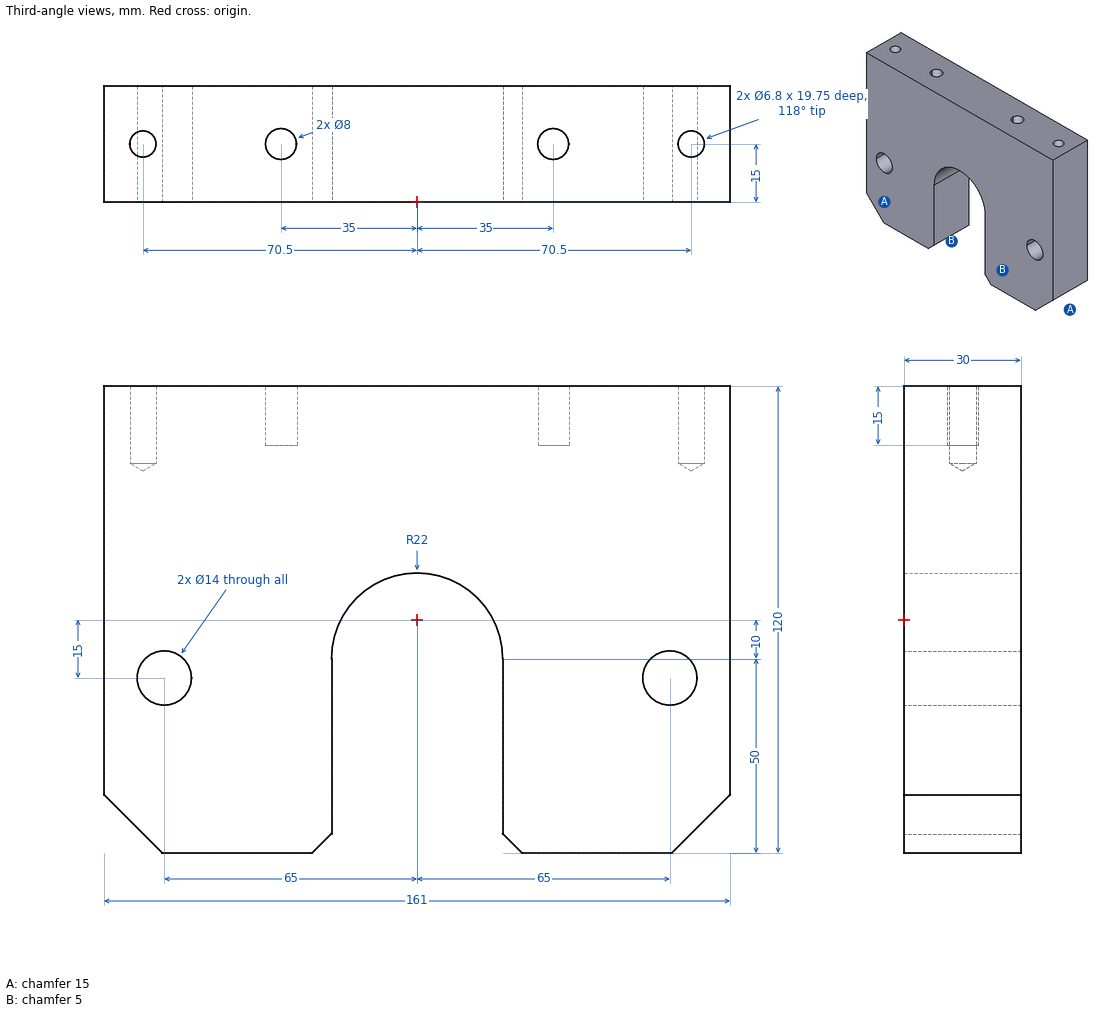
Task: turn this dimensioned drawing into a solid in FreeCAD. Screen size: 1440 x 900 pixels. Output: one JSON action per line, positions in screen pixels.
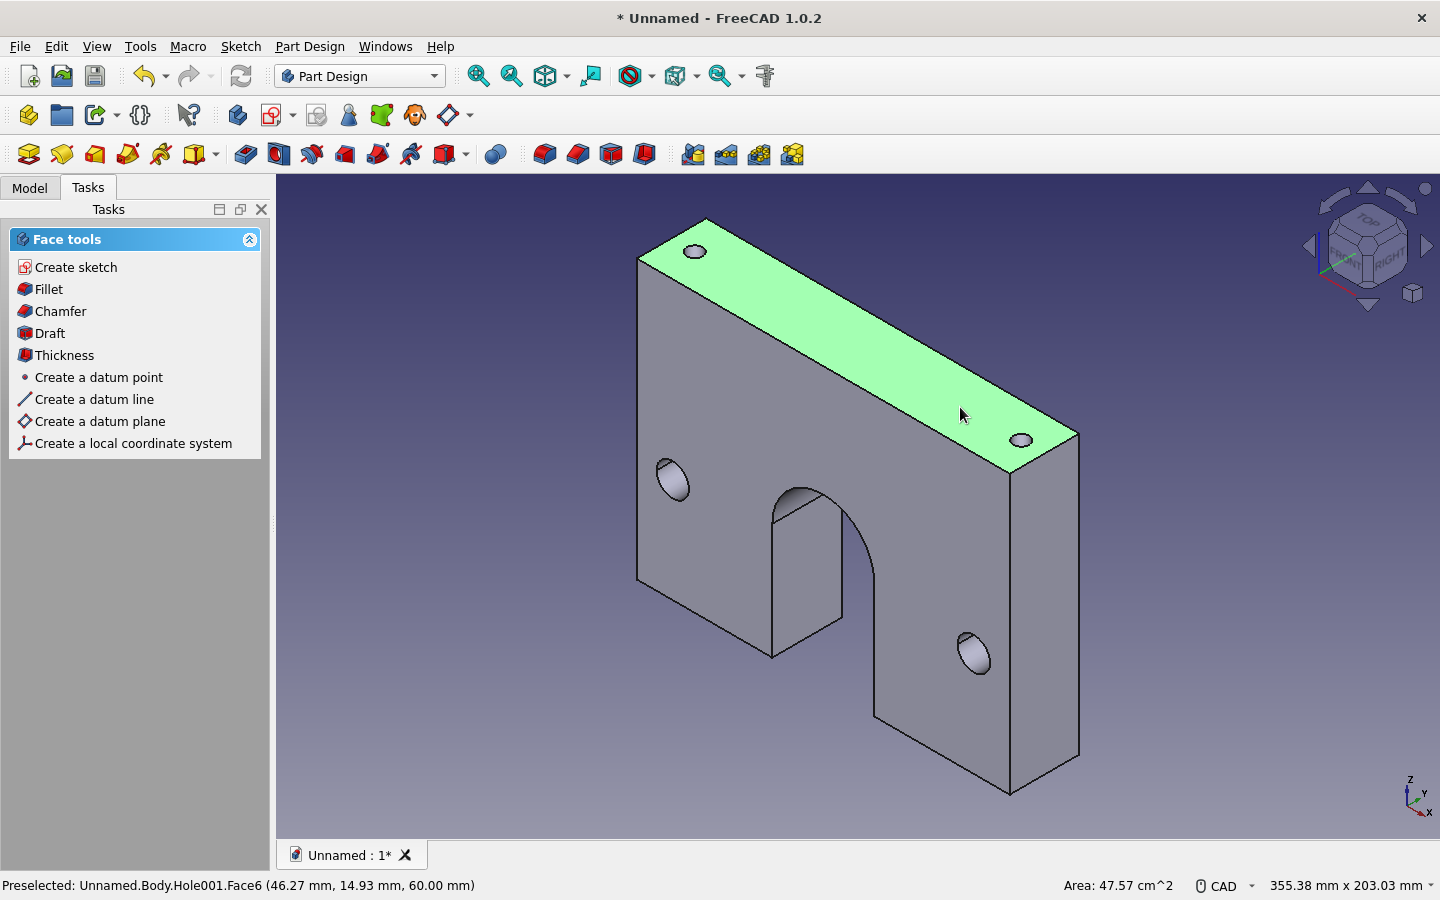
{"action": "left_click", "coordinate": [270, 116]}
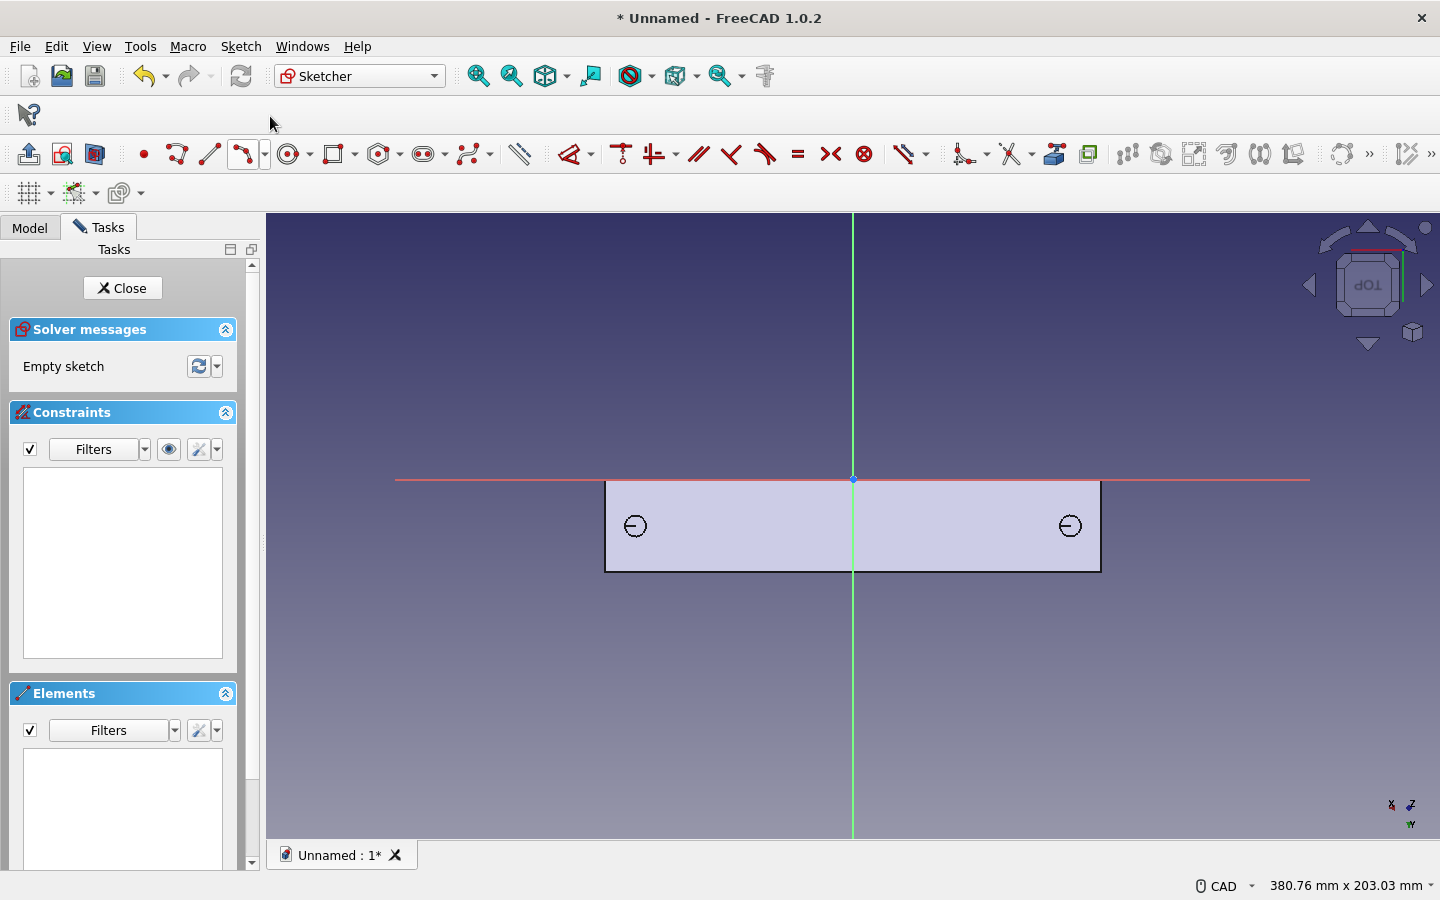
{"action": "scroll", "coordinate": [893, 499], "scroll_direction": "up", "scroll_amount": 5}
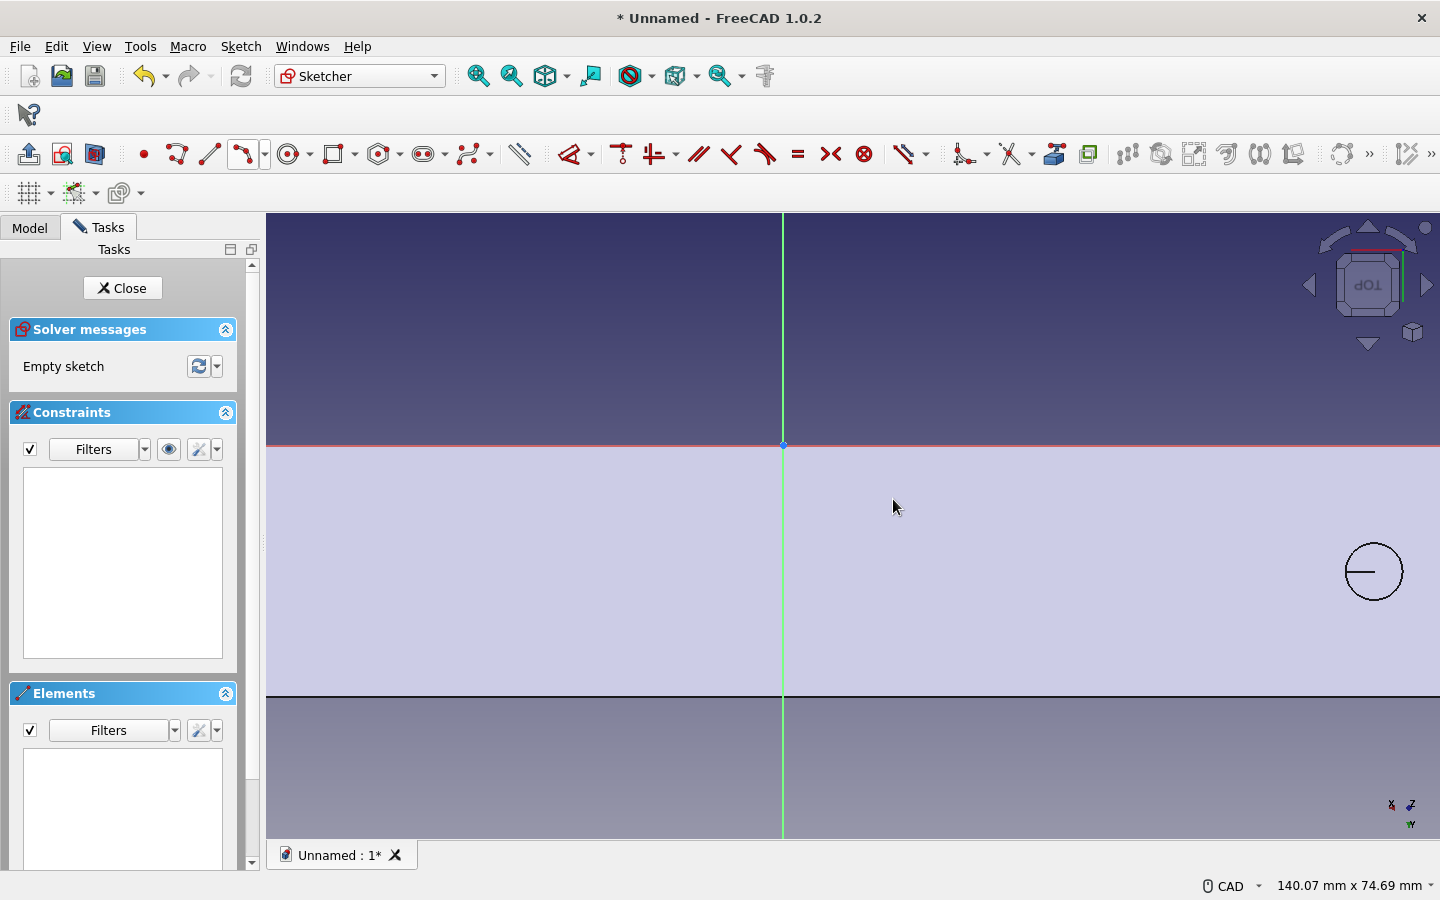
{"action": "key", "text": "g c"}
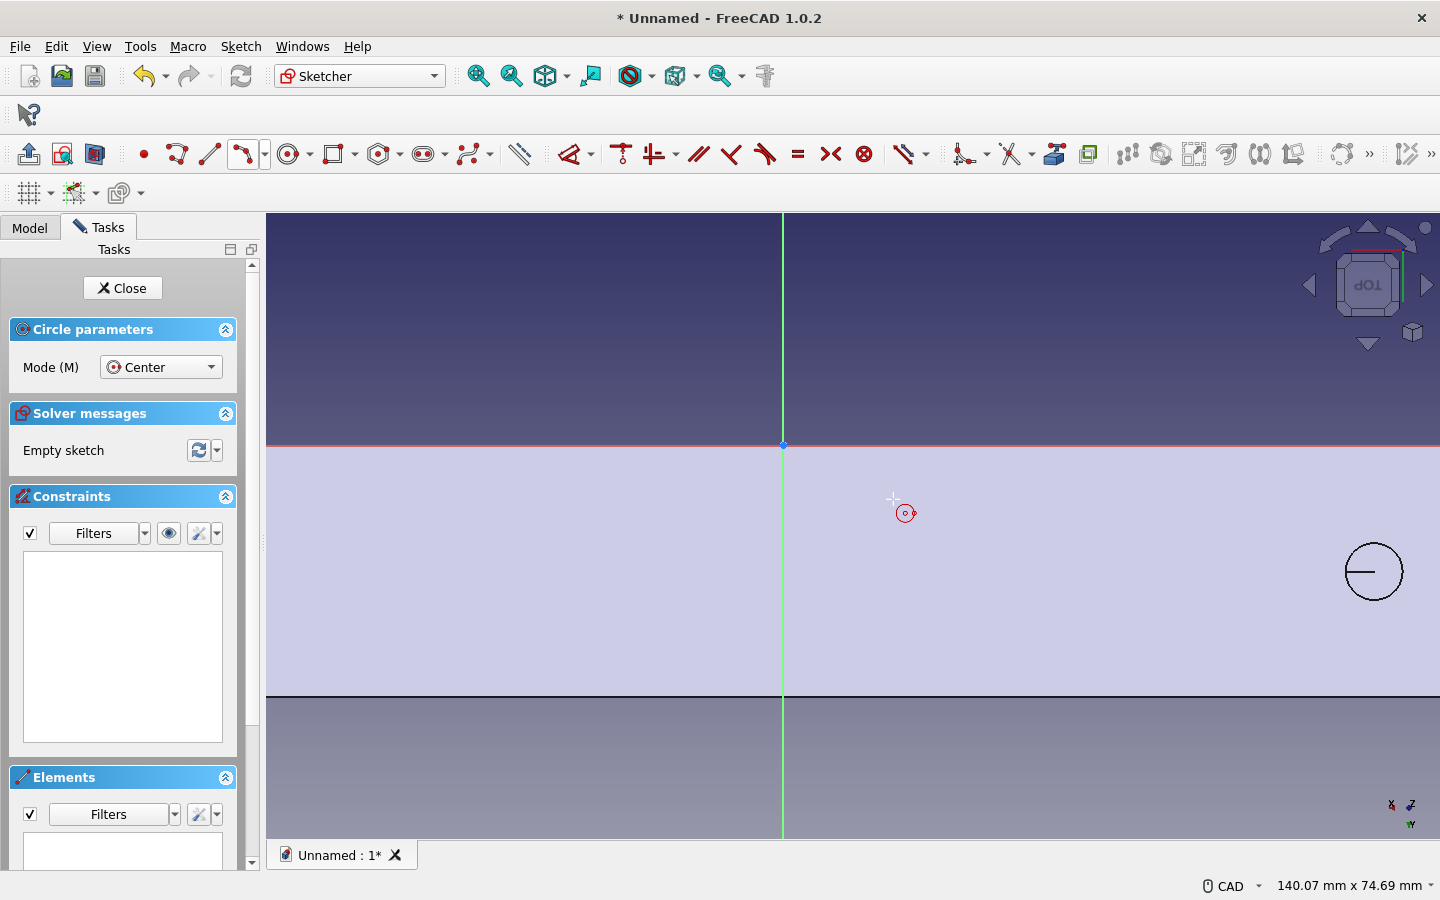
{"action": "left_click", "coordinate": [1077, 572]}
{"action": "left_click", "coordinate": [1100, 548]}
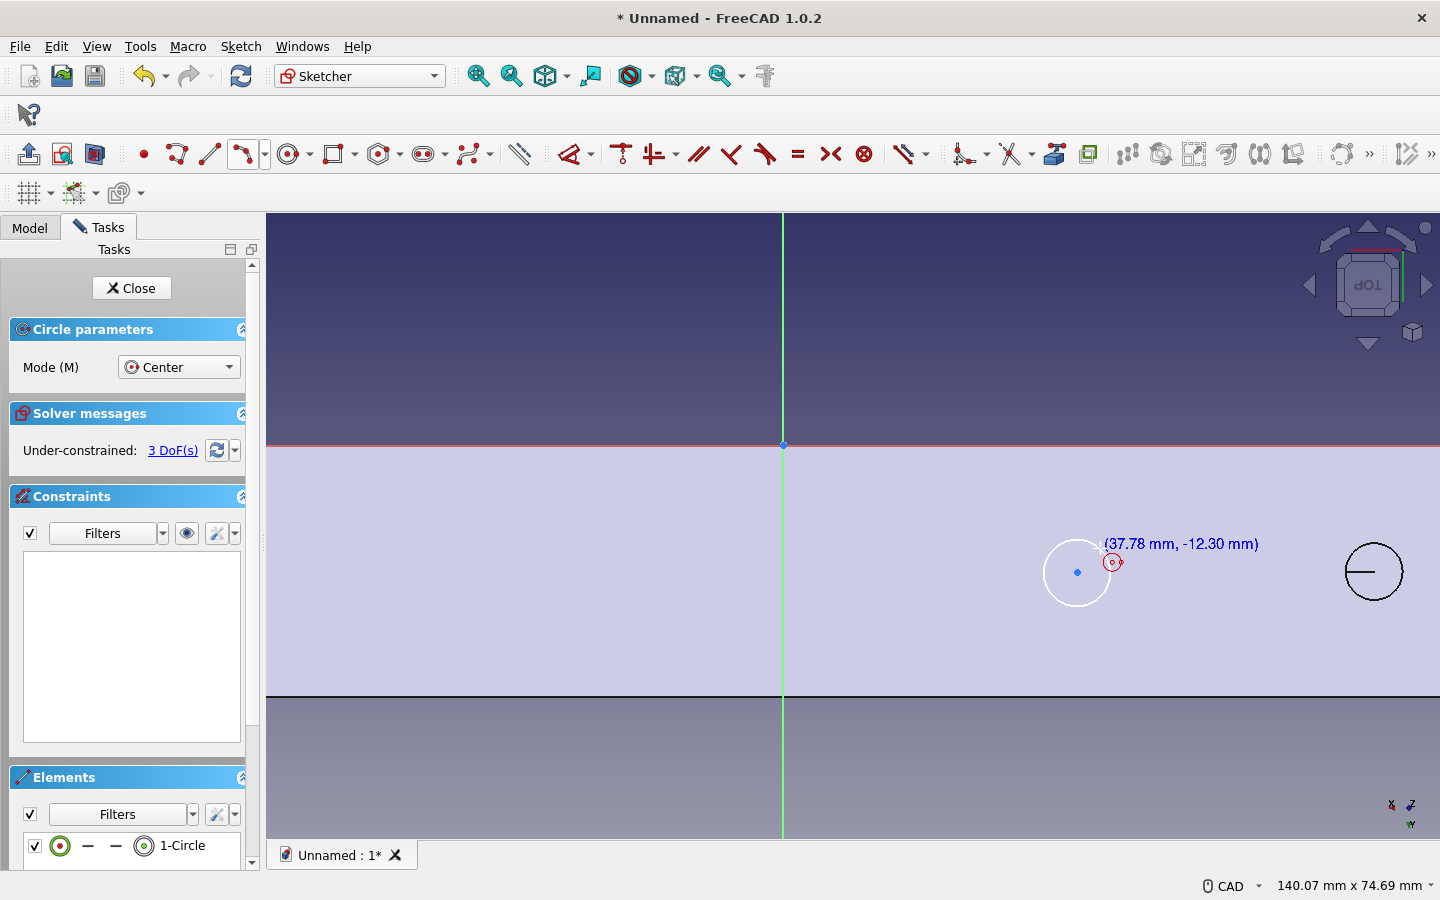
{"action": "left_click", "coordinate": [490, 572]}
{"action": "left_click", "coordinate": [514, 548]}
{"action": "key", "text": "Escape"}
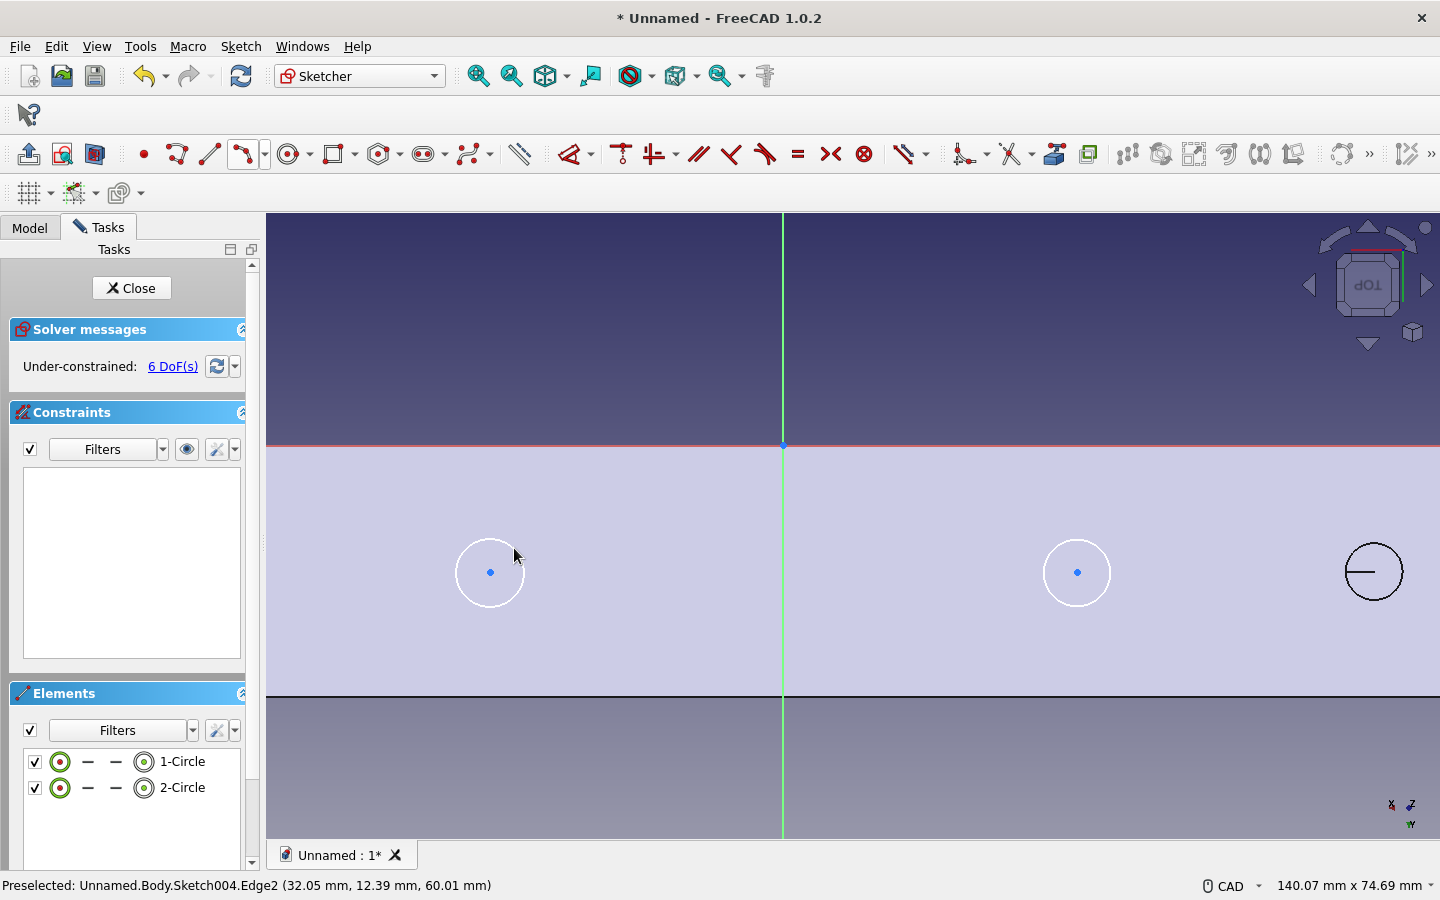
{"action": "left_click", "coordinate": [1100, 549]}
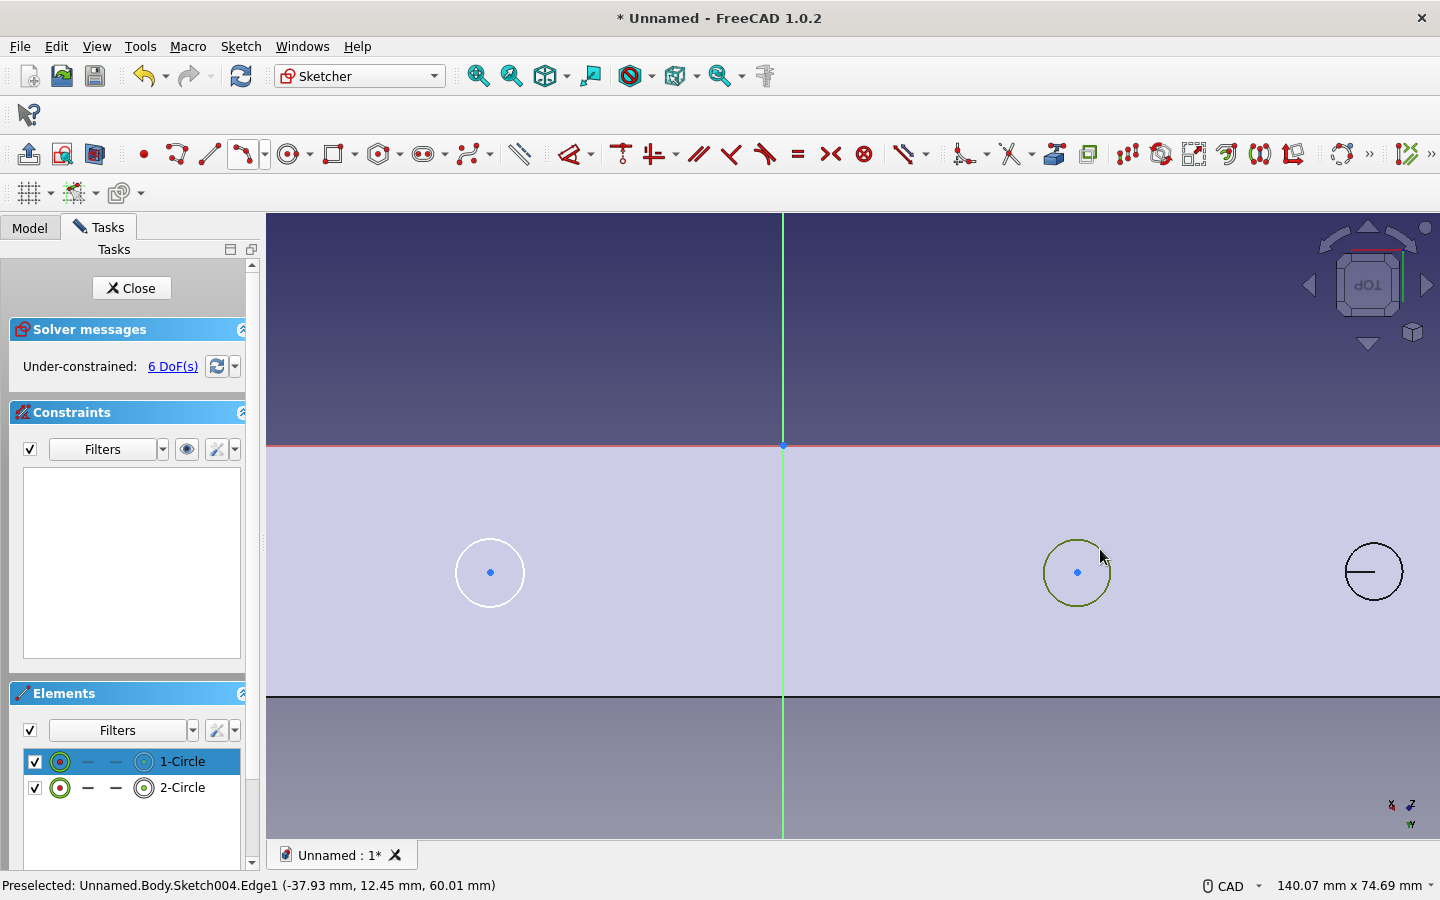
{"action": "left_click", "coordinate": [514, 549]}